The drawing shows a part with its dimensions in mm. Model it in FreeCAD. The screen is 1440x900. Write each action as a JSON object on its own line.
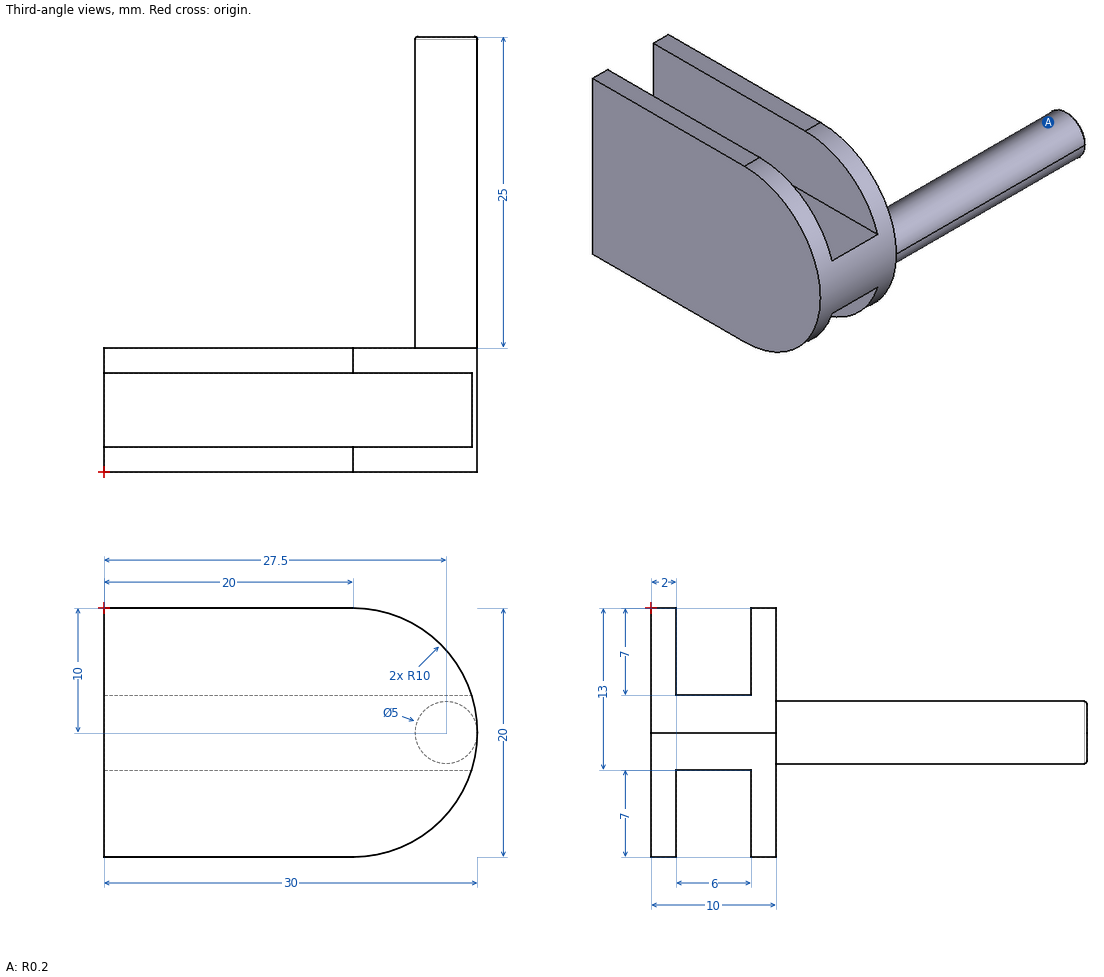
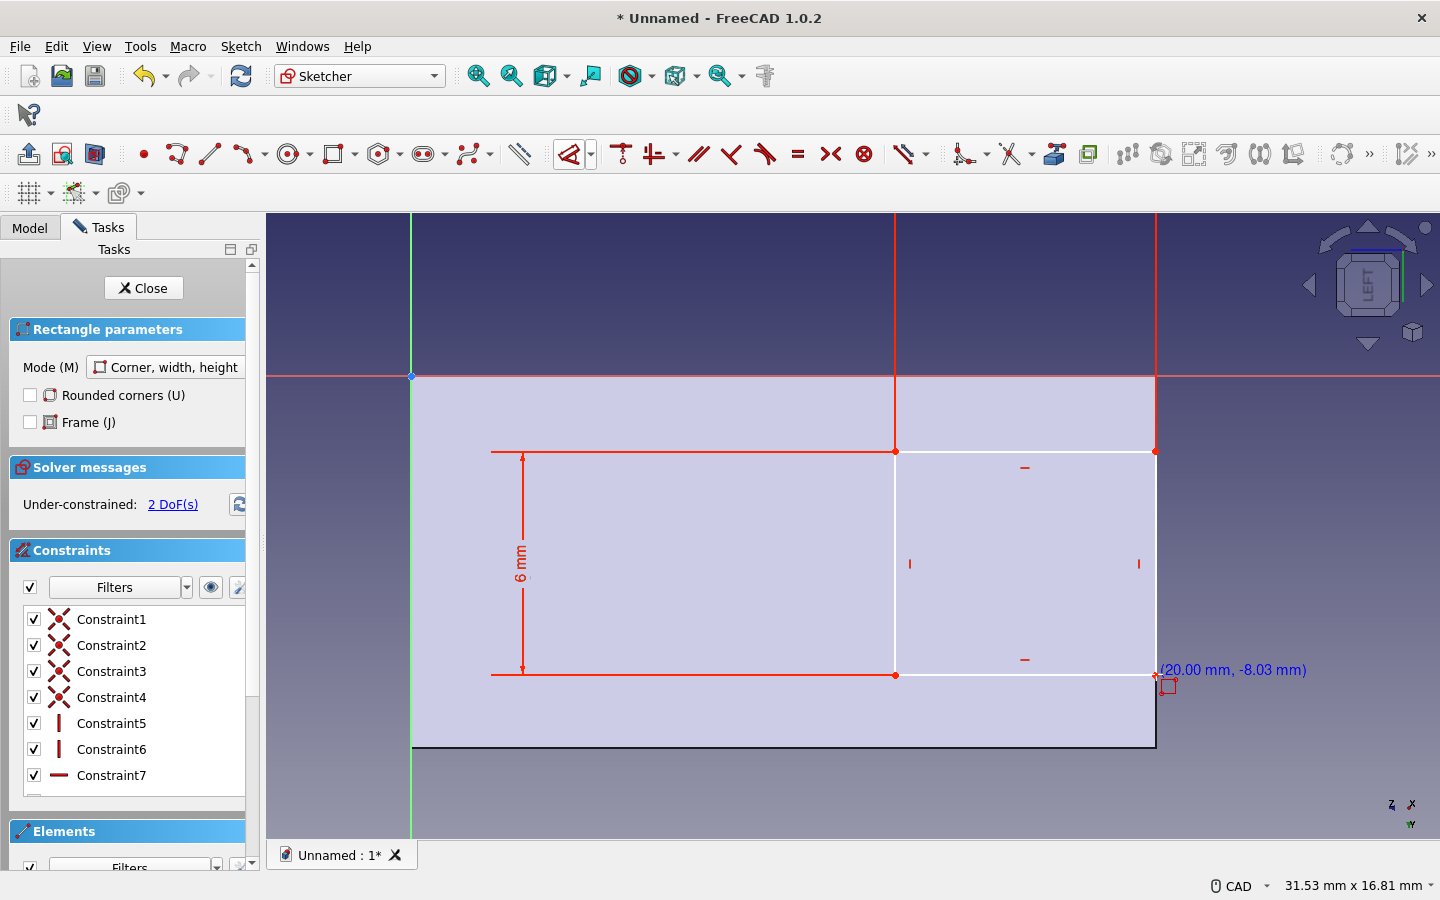
{"action": "left_click", "coordinate": [411, 451]}
{"action": "mouse_move", "coordinate": [672, 674]}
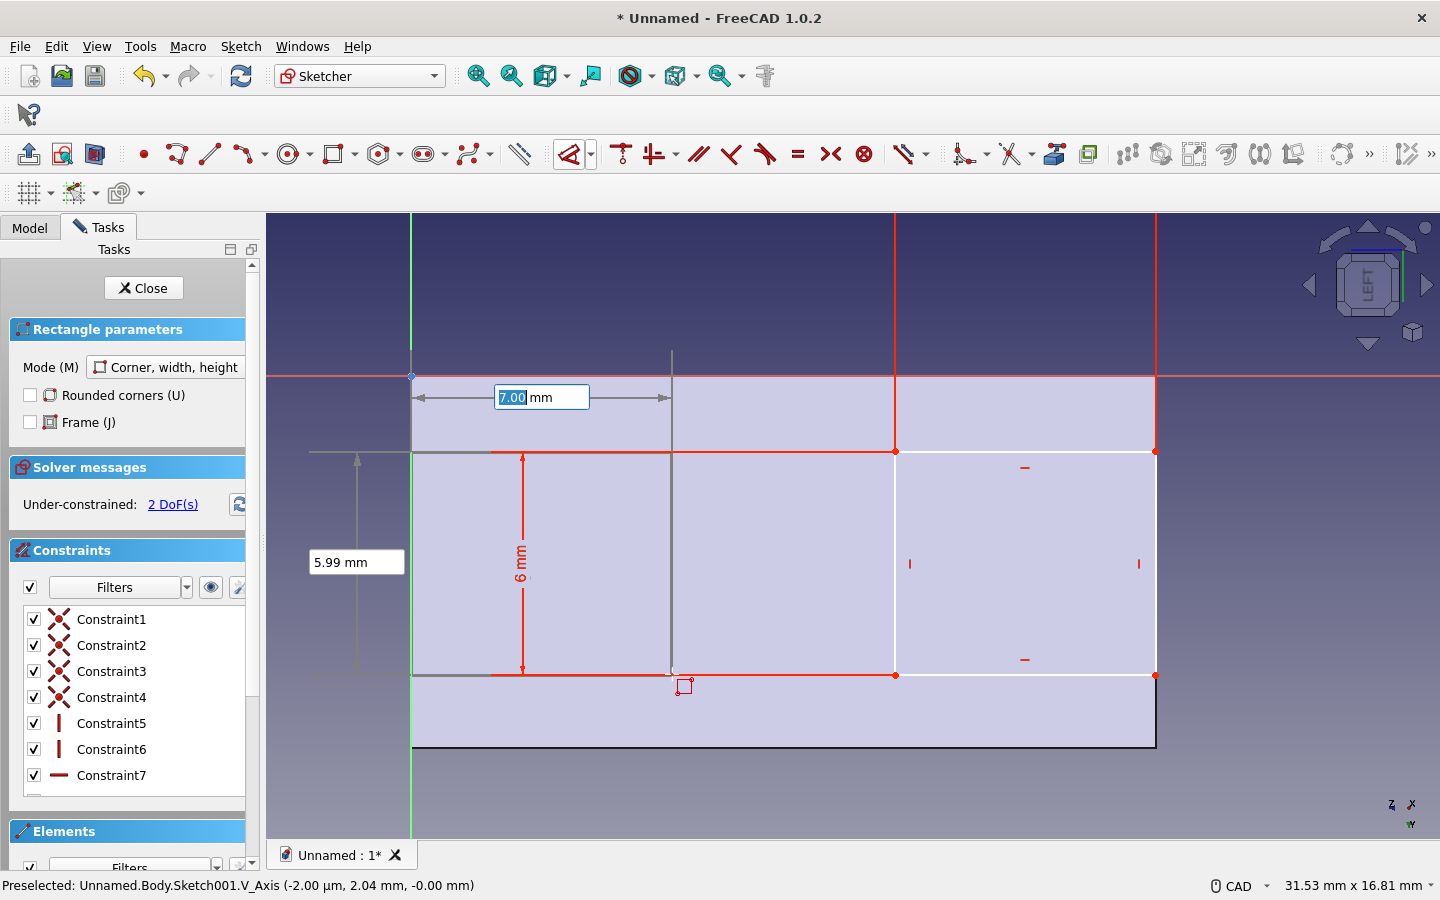
{"action": "type", "text": "7"}
{"action": "key", "text": "Tab"}
{"action": "type", "text": "6"}
{"action": "key", "text": "Return"}
{"action": "key", "text": "Escape"}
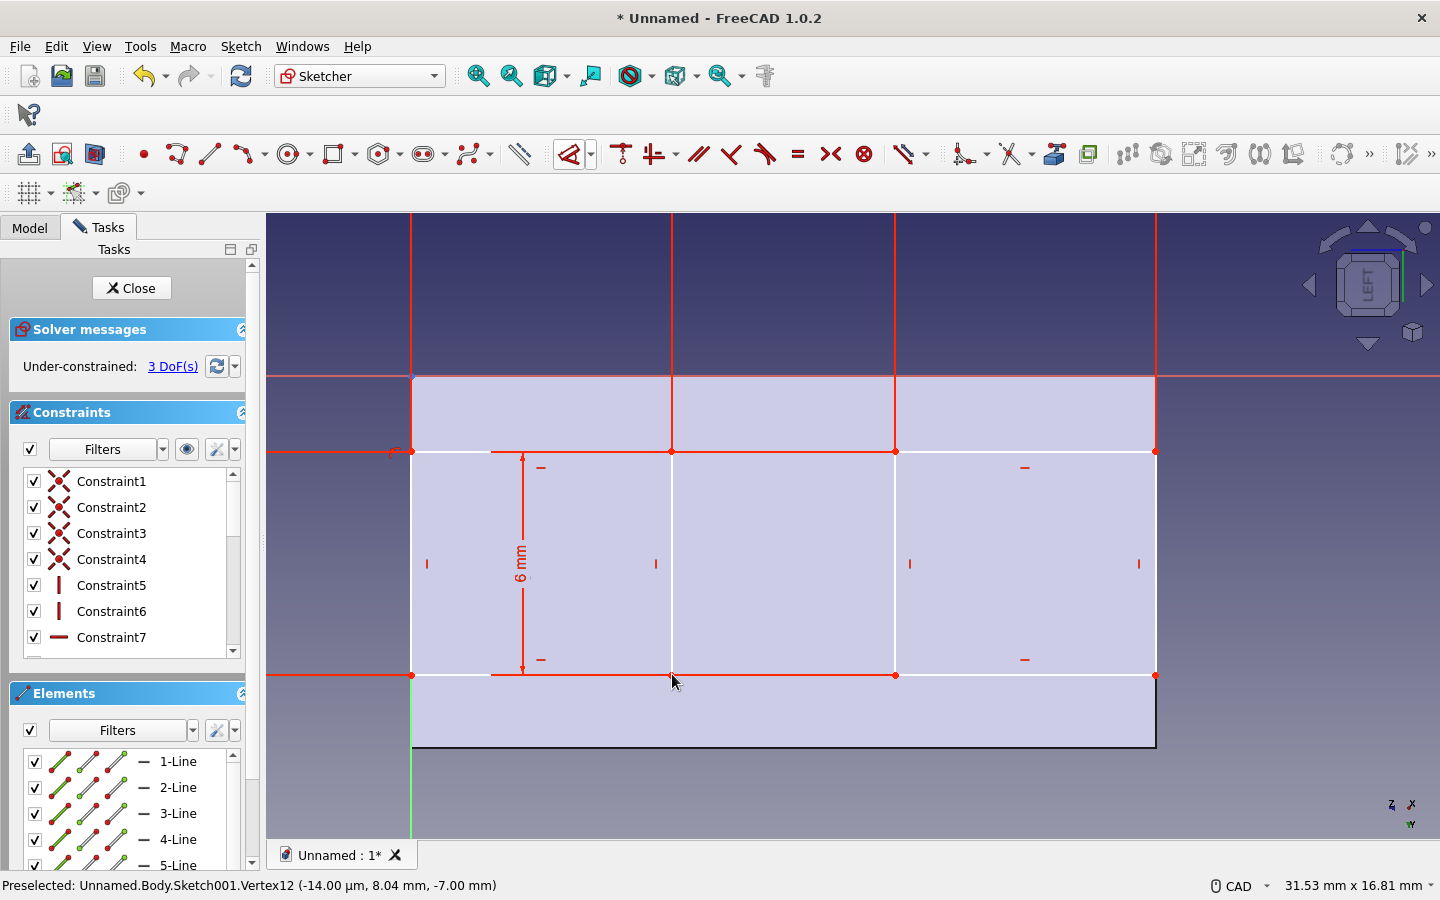
{"action": "left_click", "coordinate": [895, 452]}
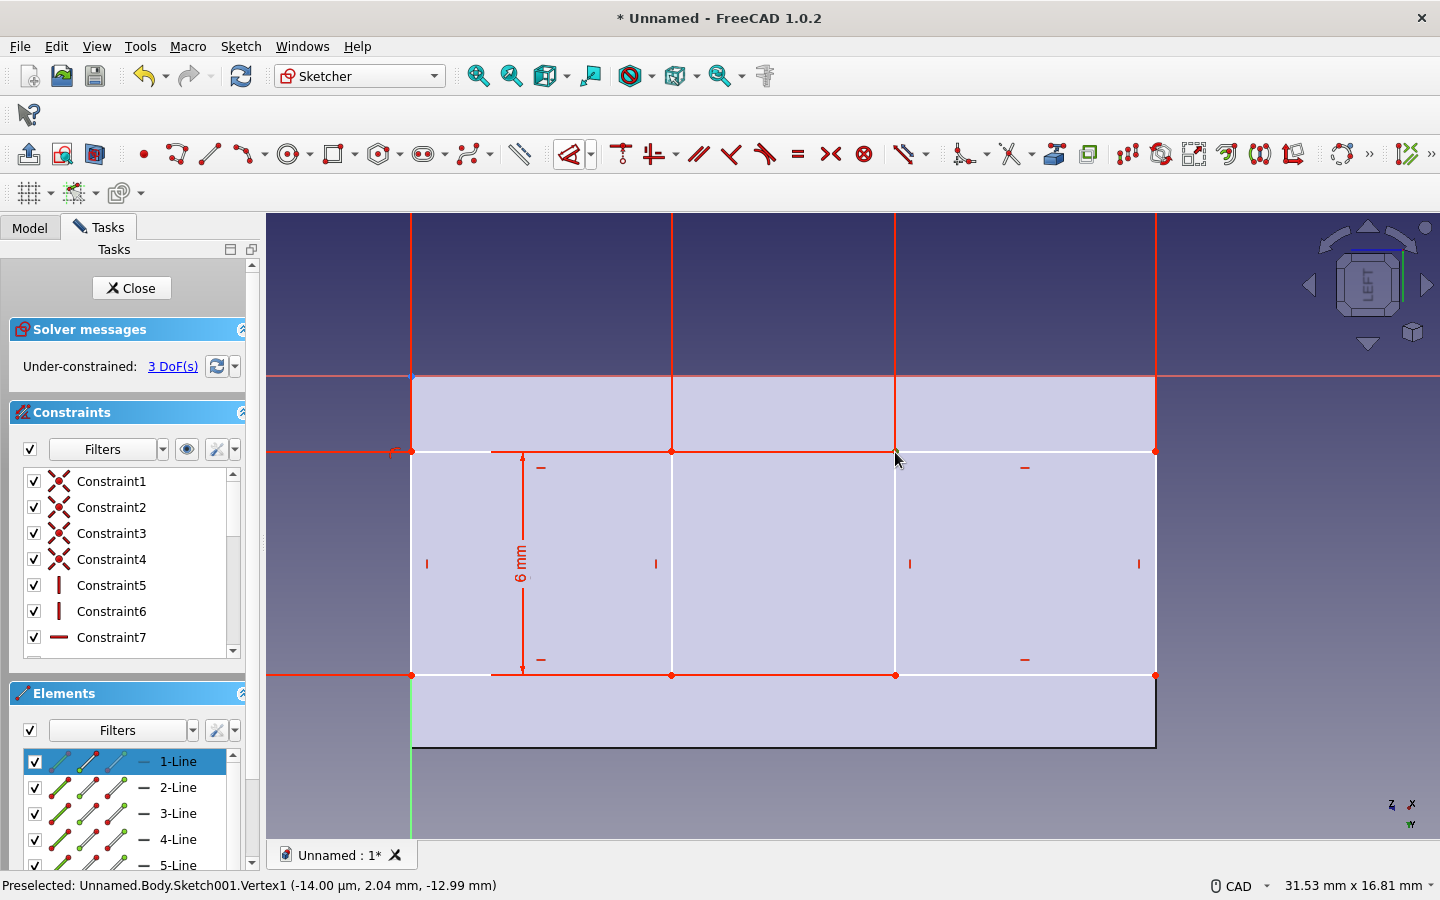
{"action": "left_click", "coordinate": [590, 154]}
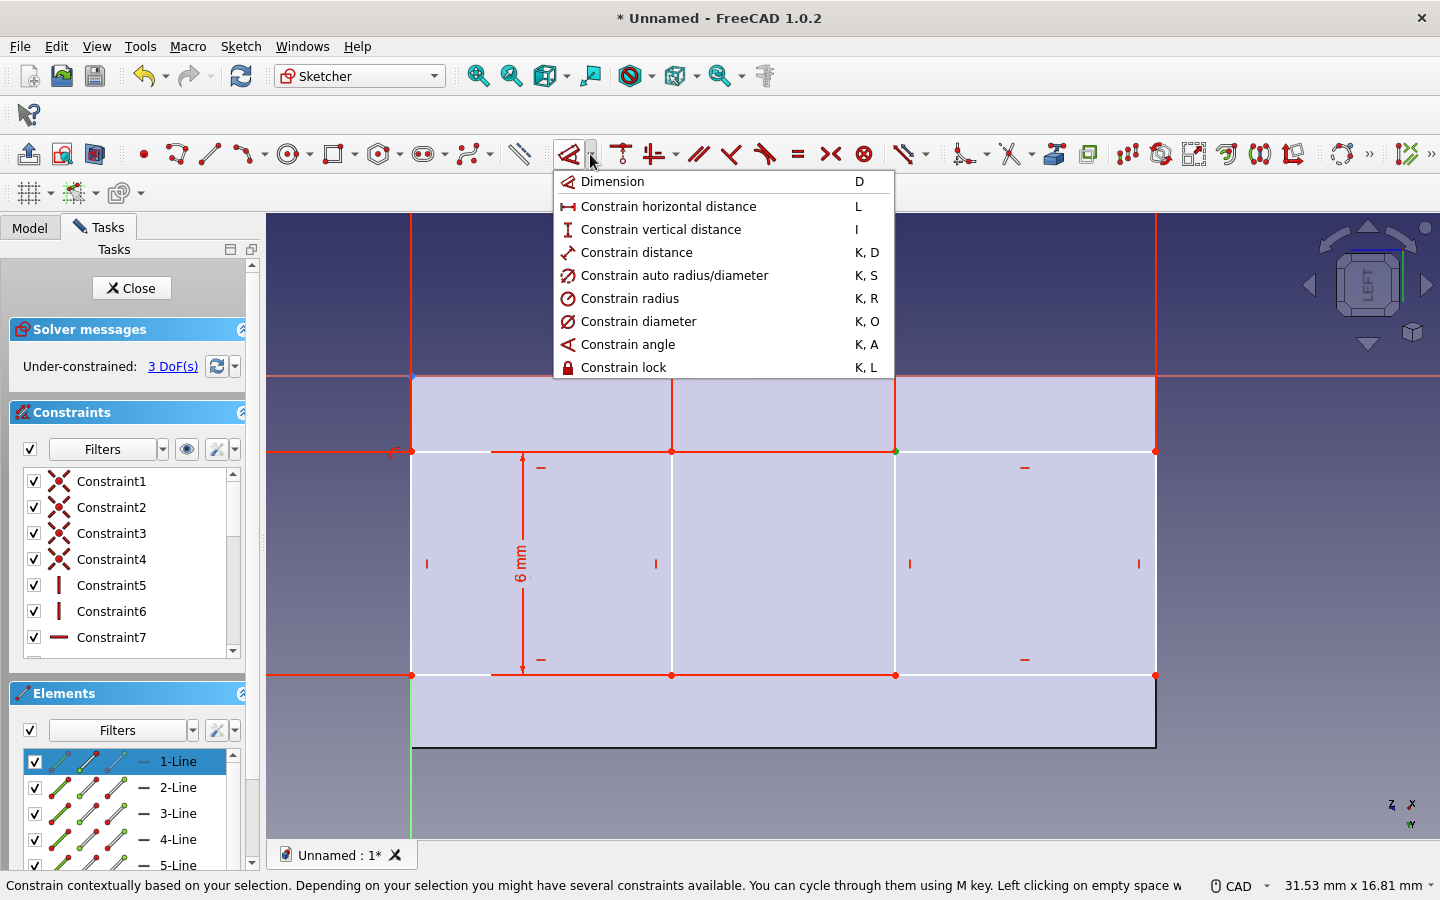
{"action": "left_click", "coordinate": [724, 230]}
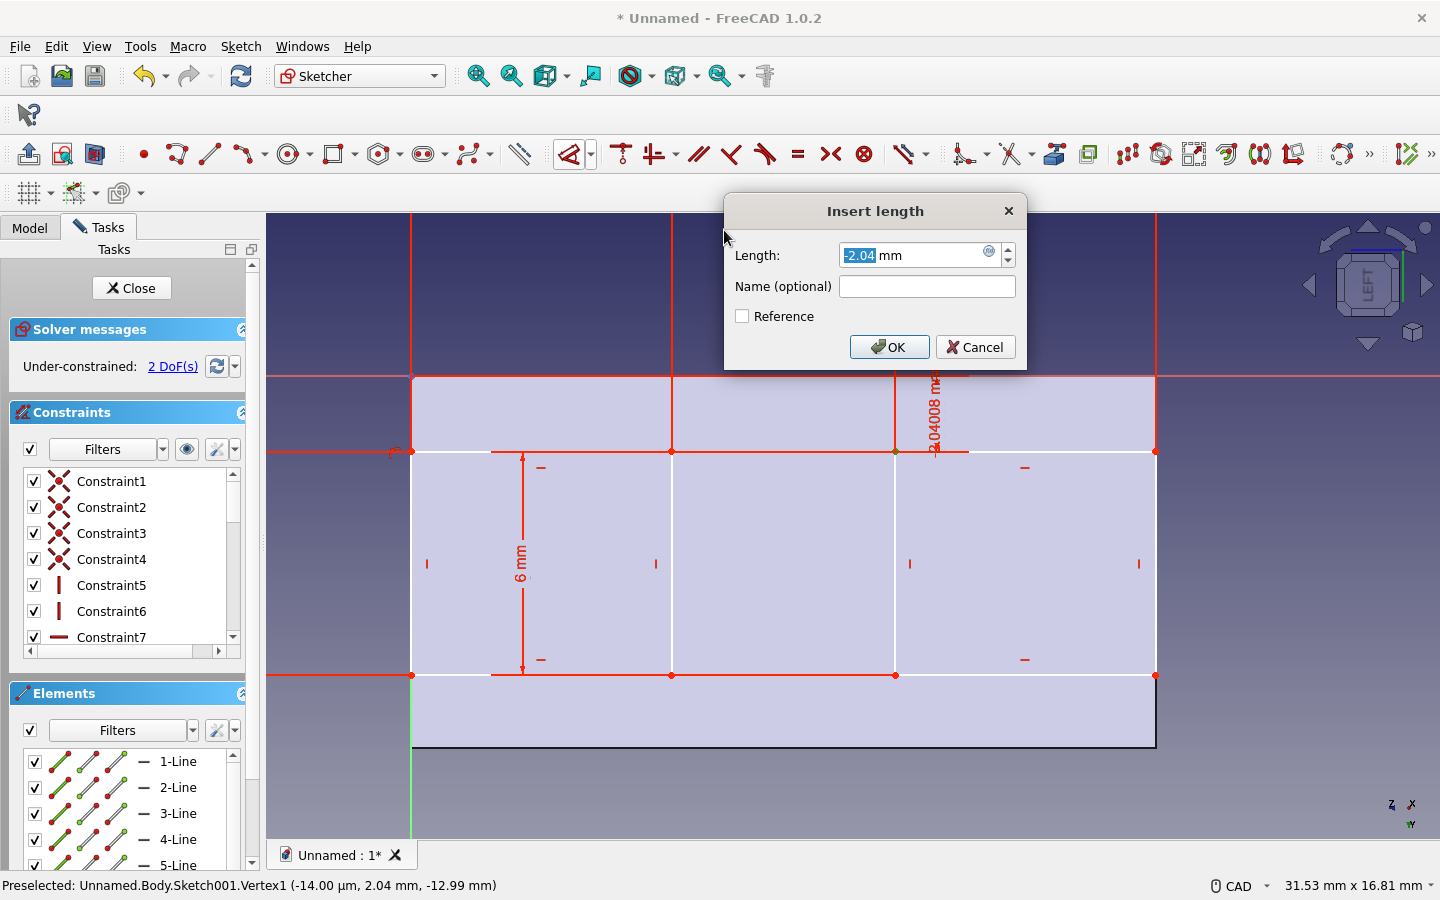
{"action": "type", "text": "-2"}
{"action": "key", "text": "Return"}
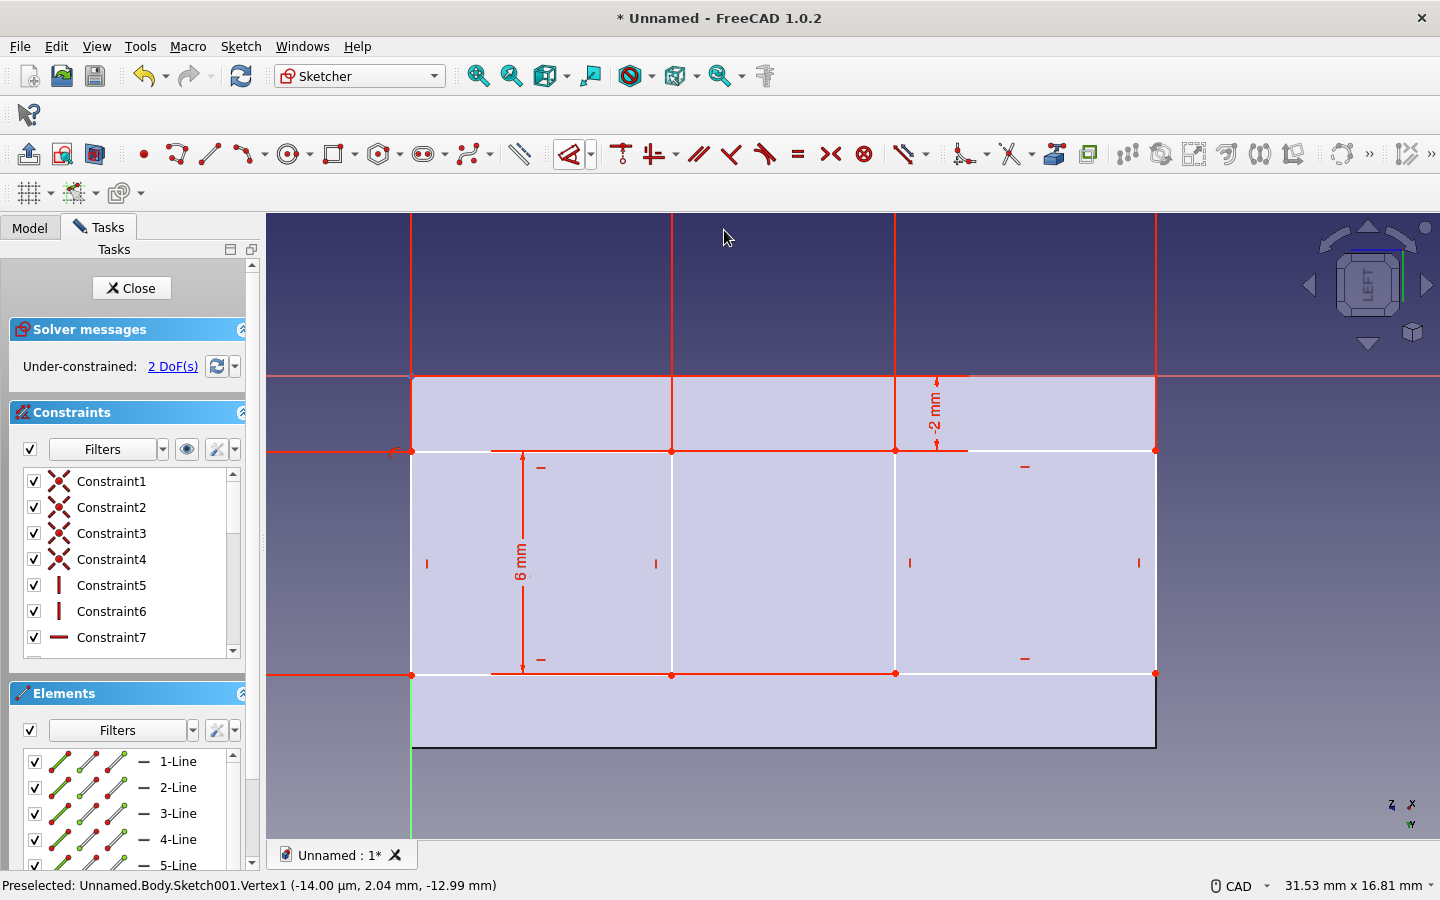
{"action": "left_click", "coordinate": [411, 452]}